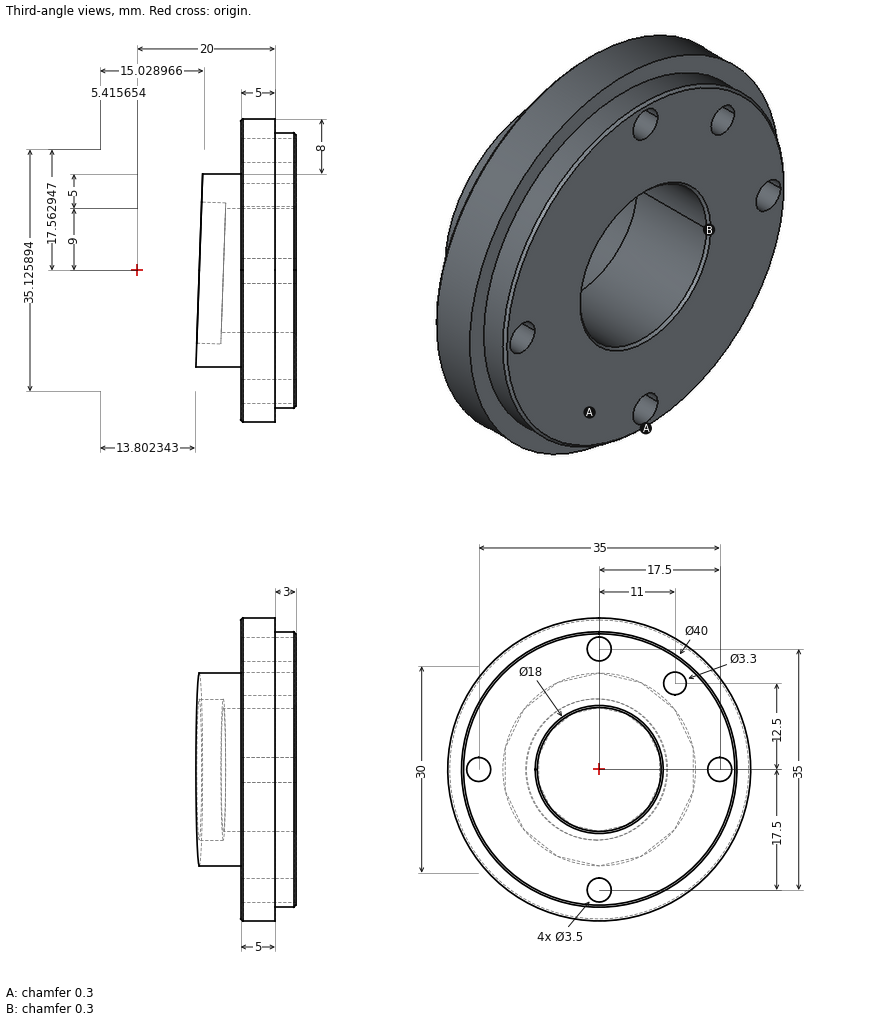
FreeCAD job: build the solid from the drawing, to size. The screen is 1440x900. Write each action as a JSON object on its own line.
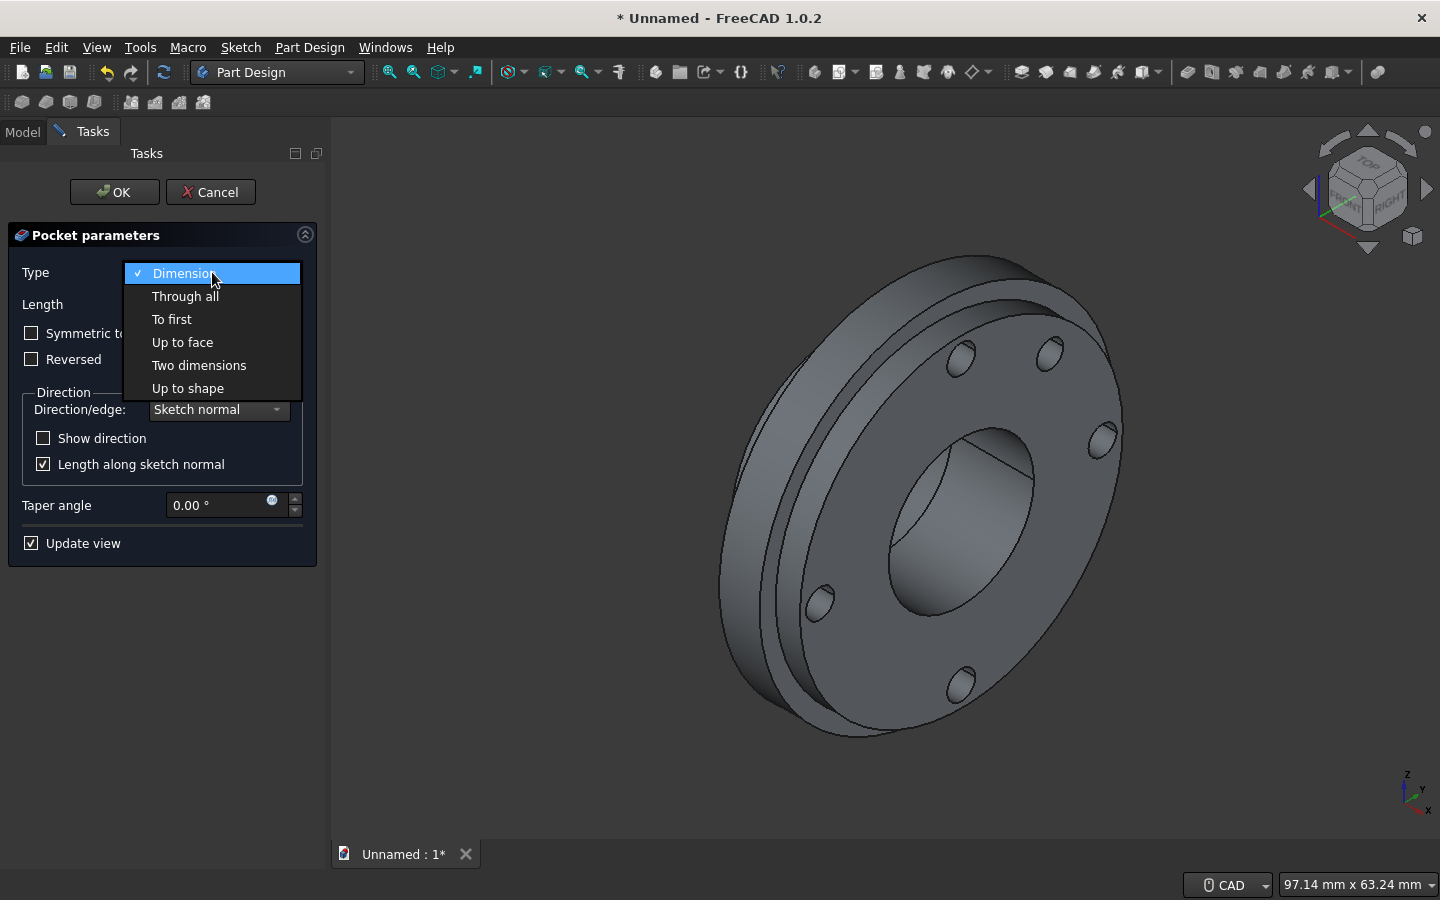
{"action": "left_click", "coordinate": [212, 320]}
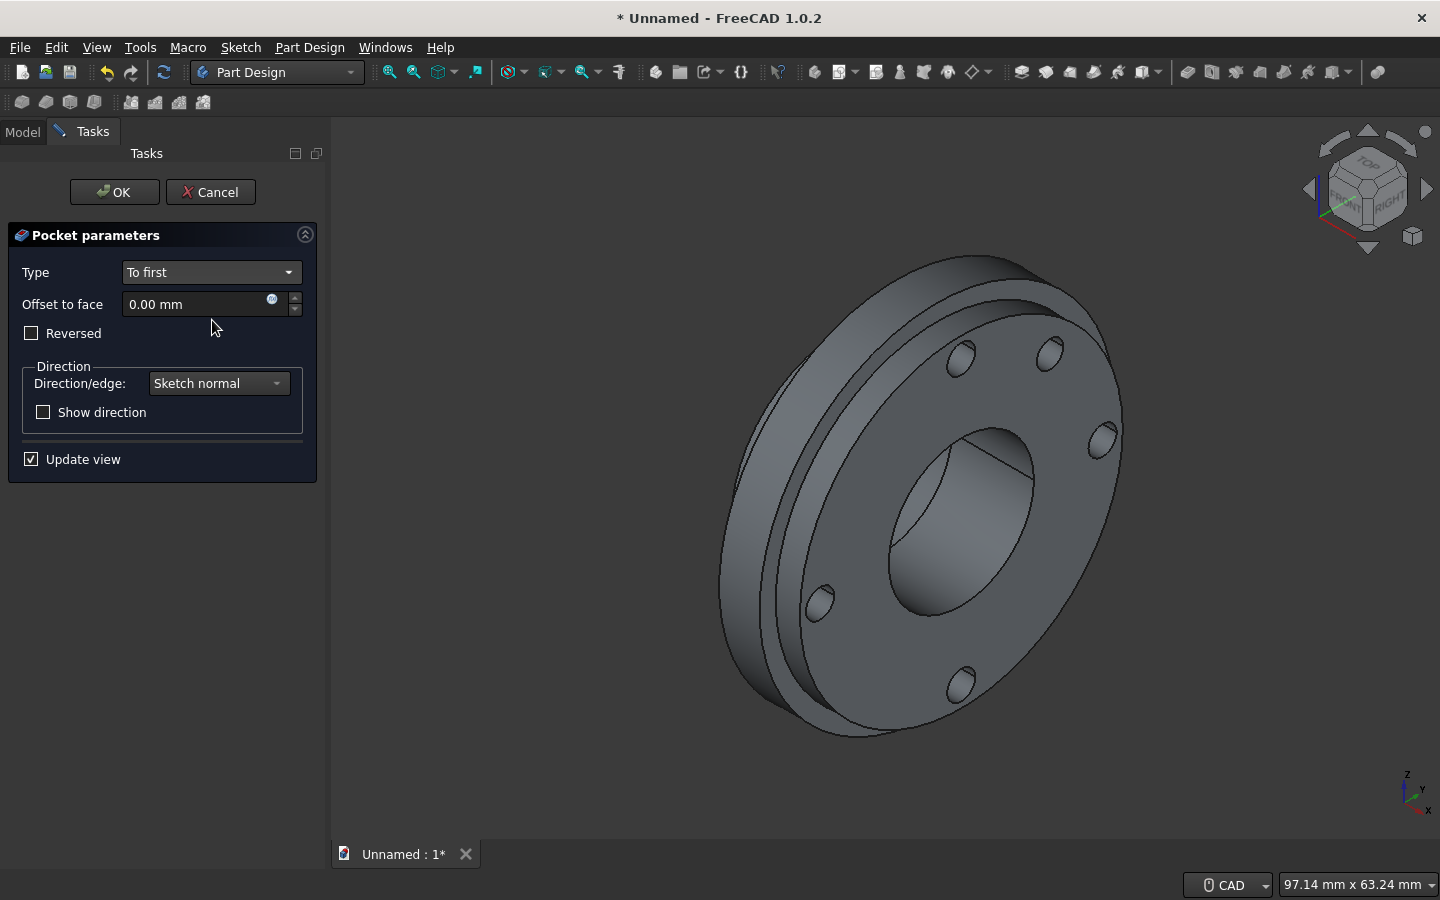
{"action": "left_click", "coordinate": [115, 192]}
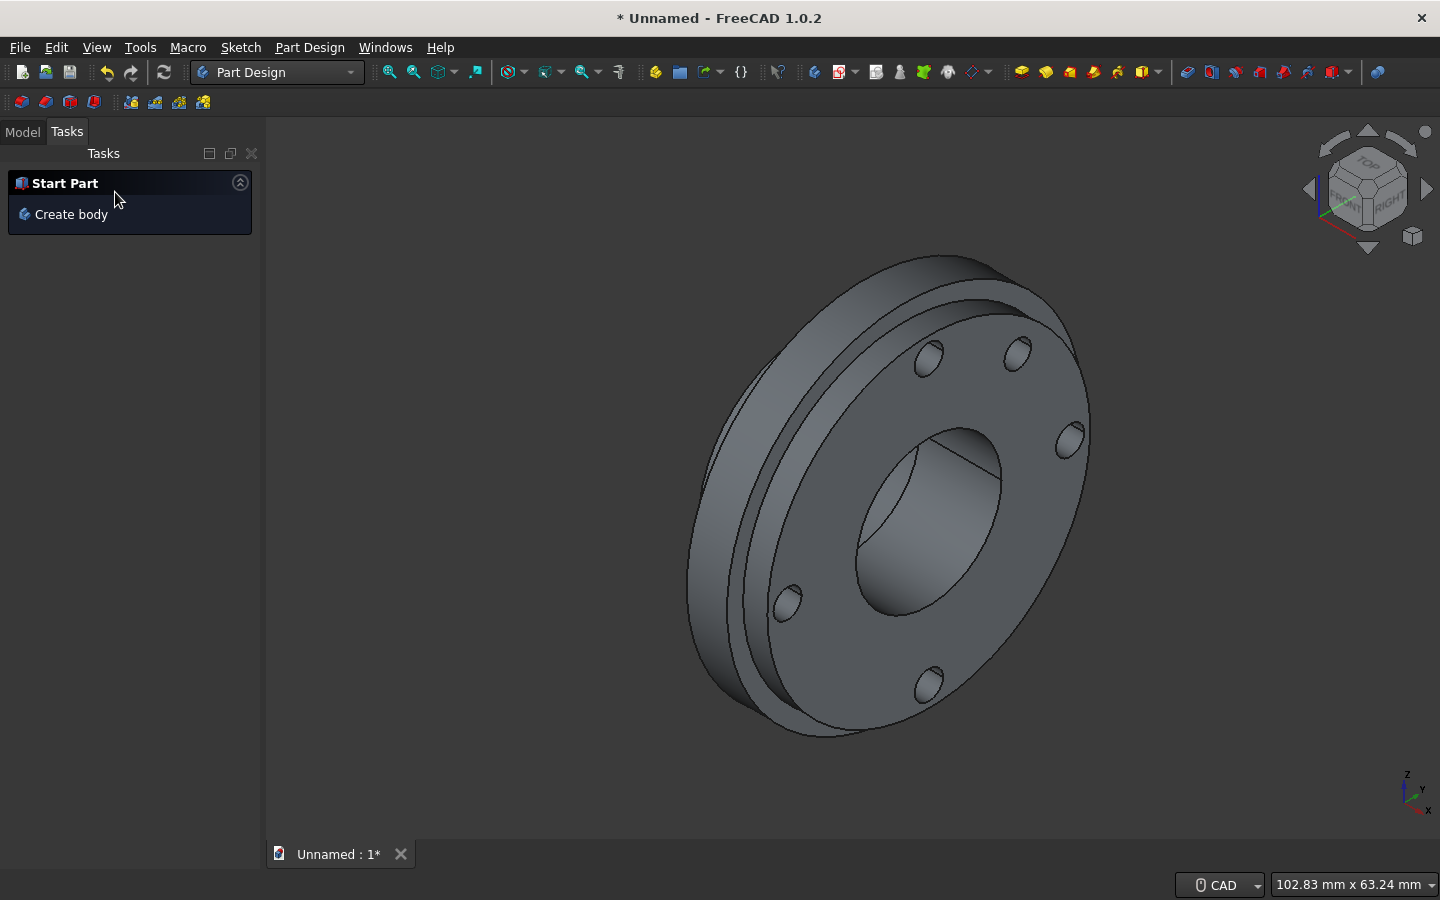
{"action": "left_click", "coordinate": [767, 614]}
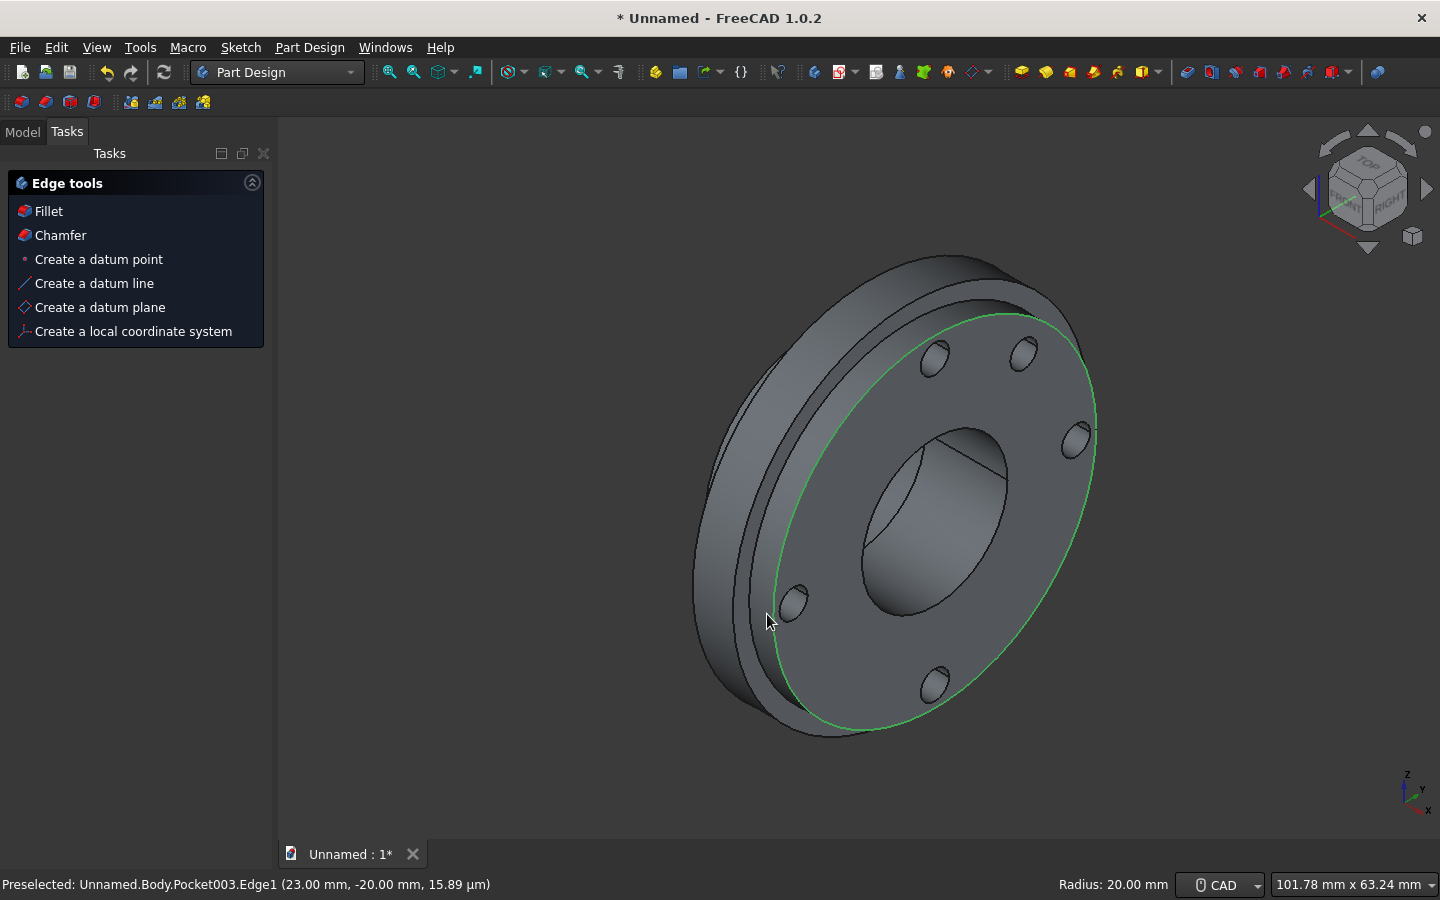
{"action": "key", "text": "2"}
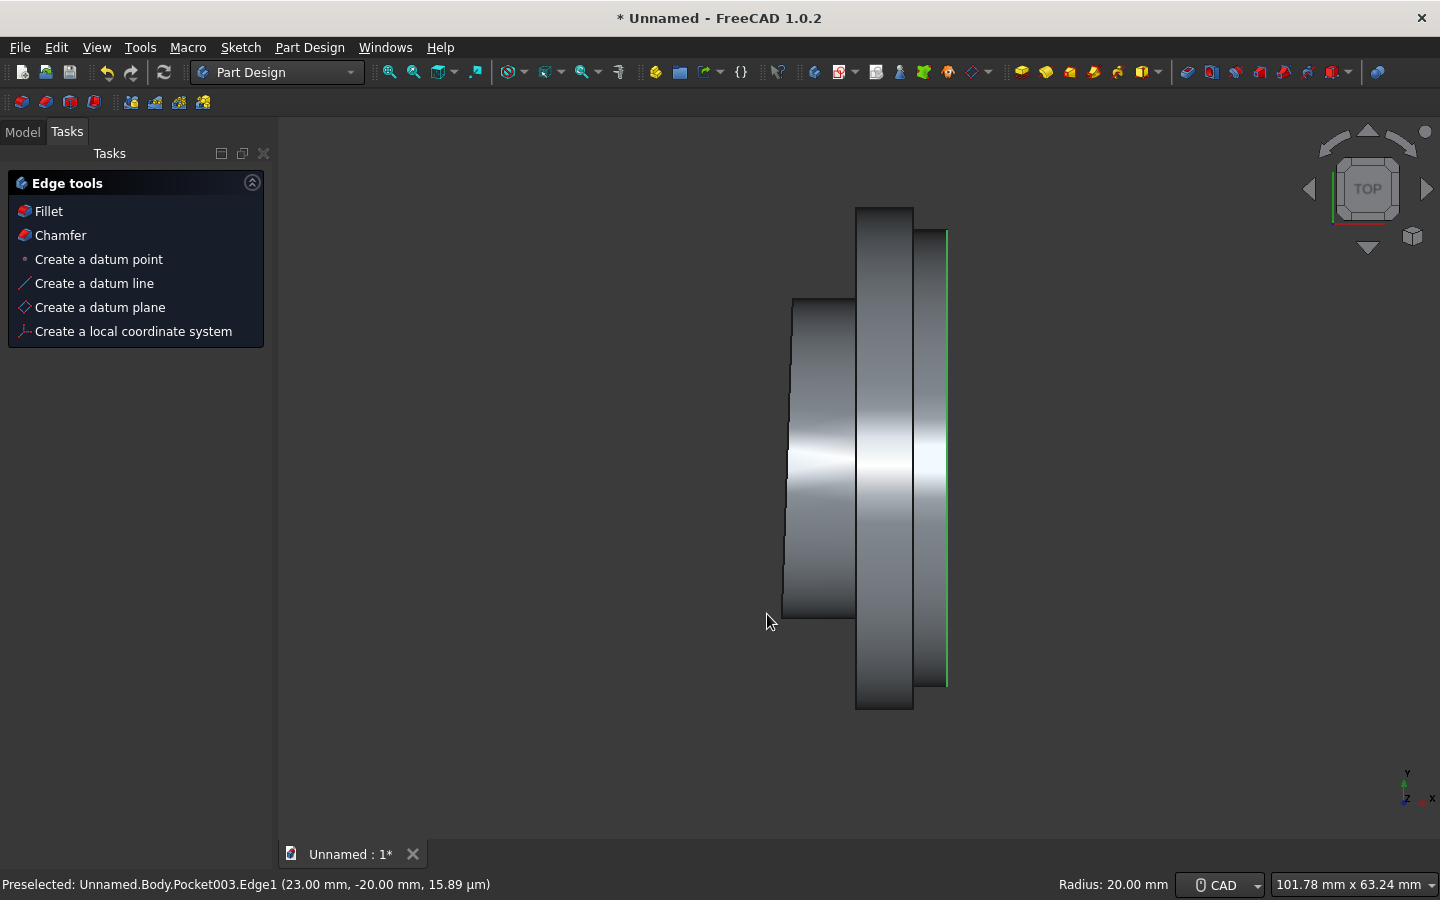
{"action": "left_click", "coordinate": [856, 661], "text": "ctrl"}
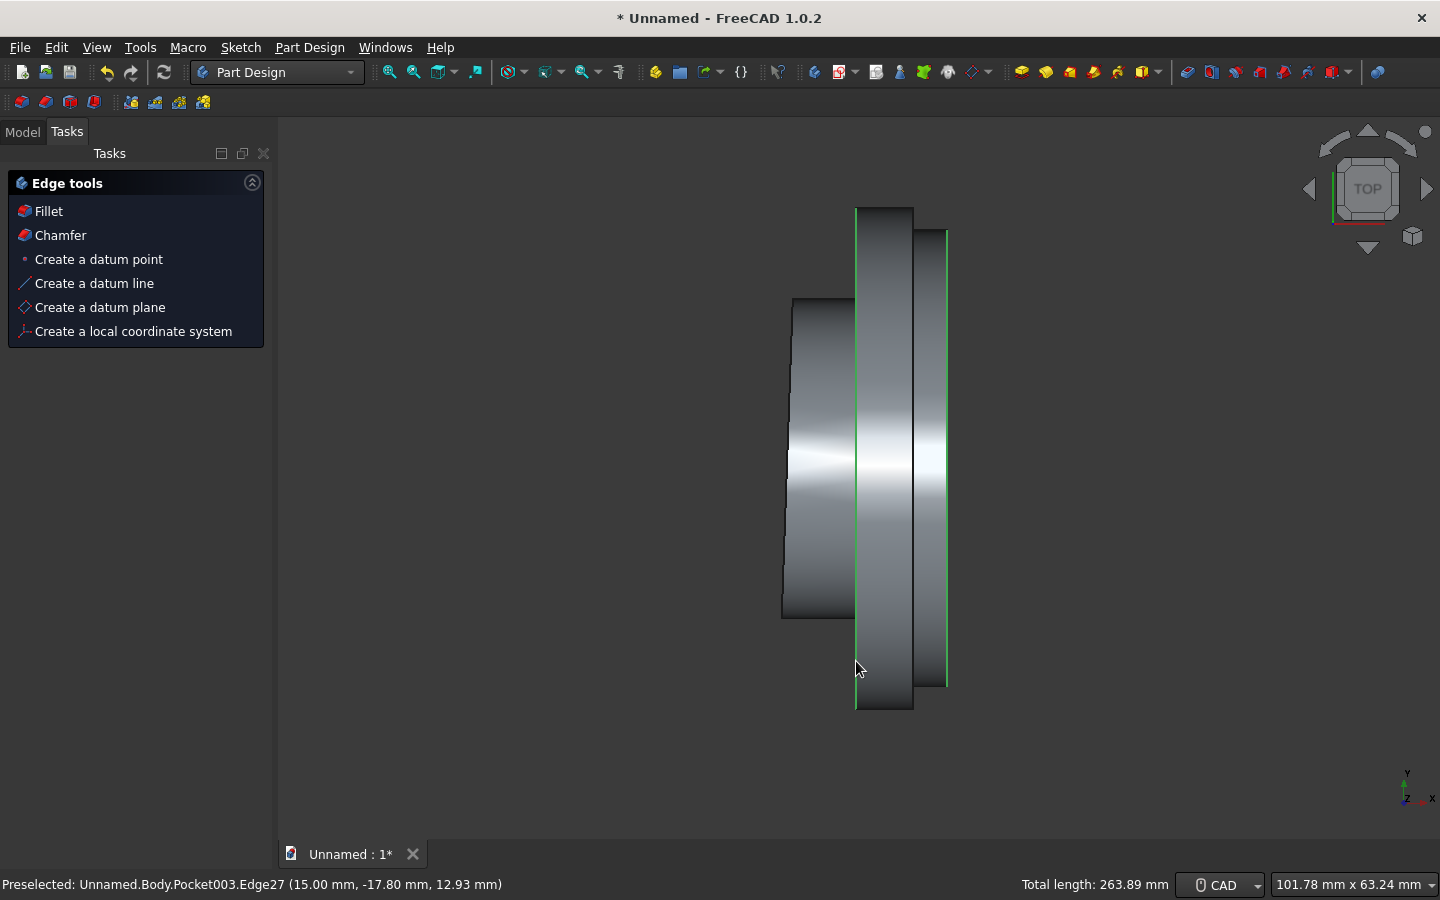
{"action": "left_click", "coordinate": [46, 102]}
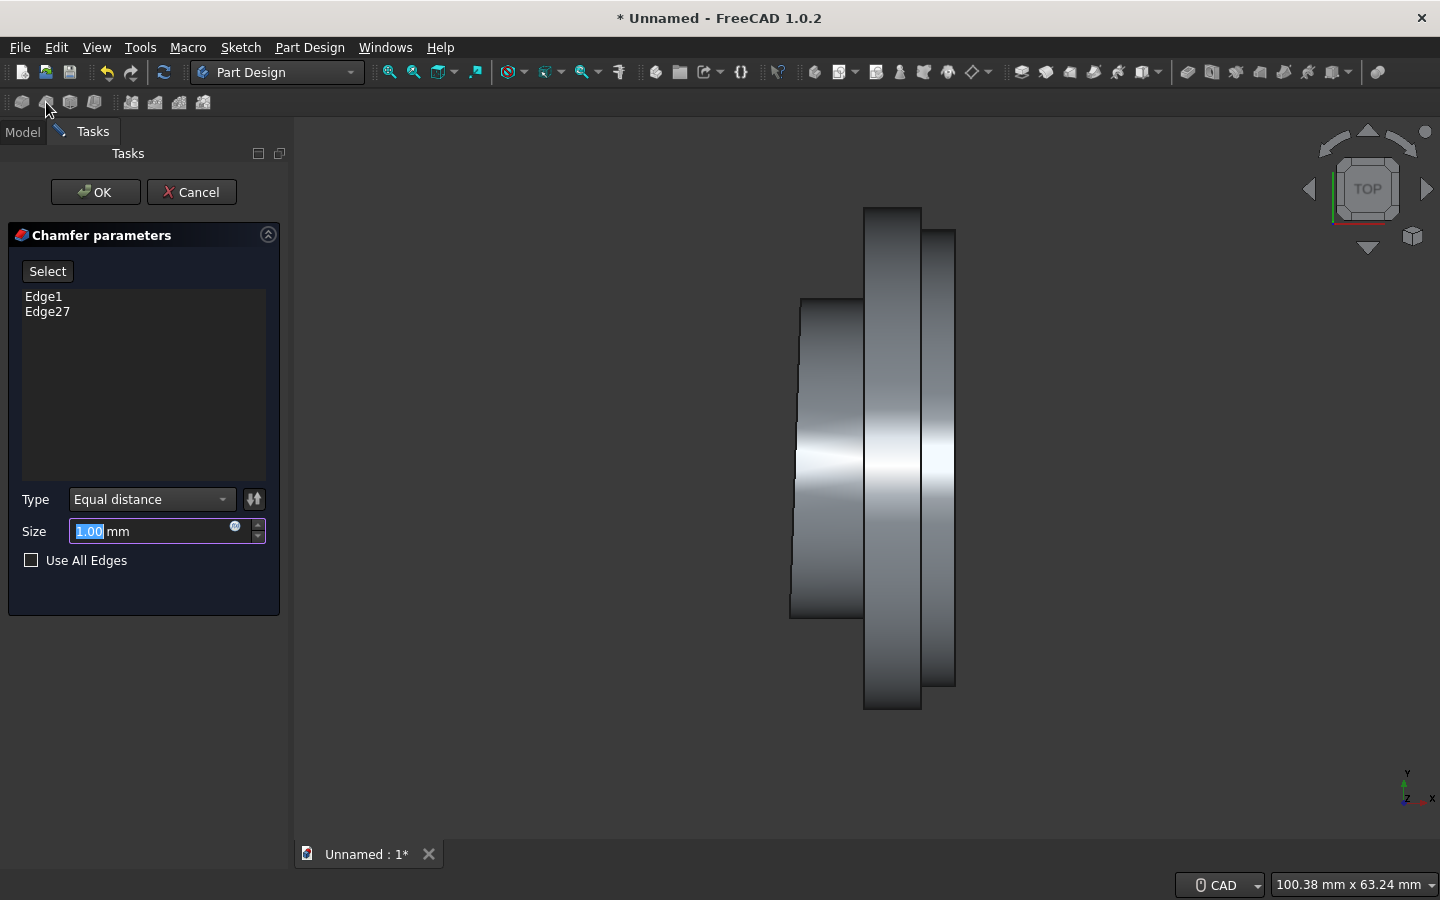
{"action": "type", "text": "0.3"}
{"action": "key", "text": "Tab"}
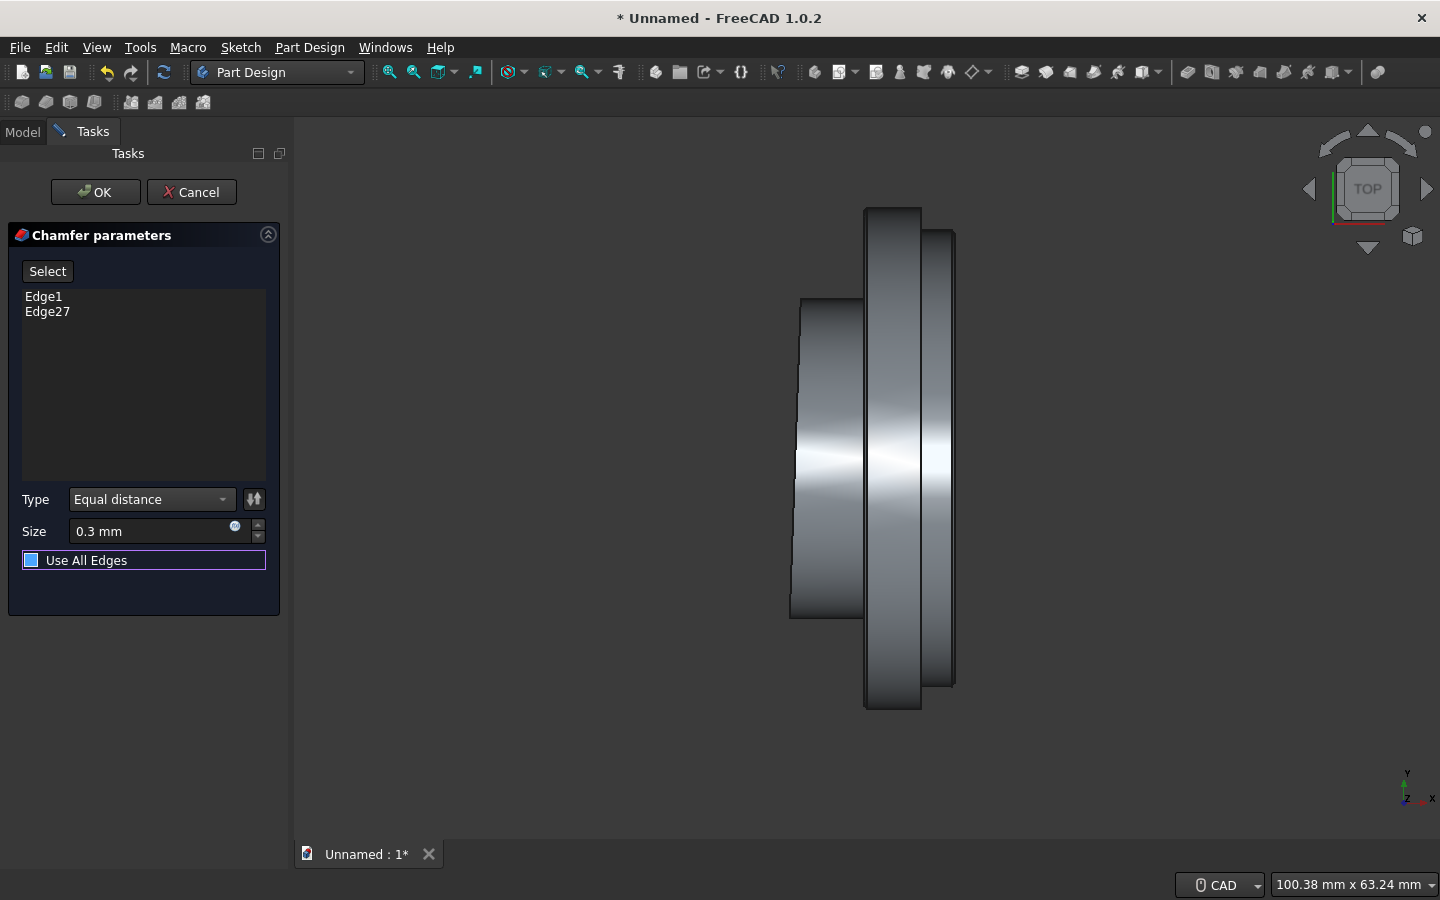
{"action": "left_click", "coordinate": [96, 192]}